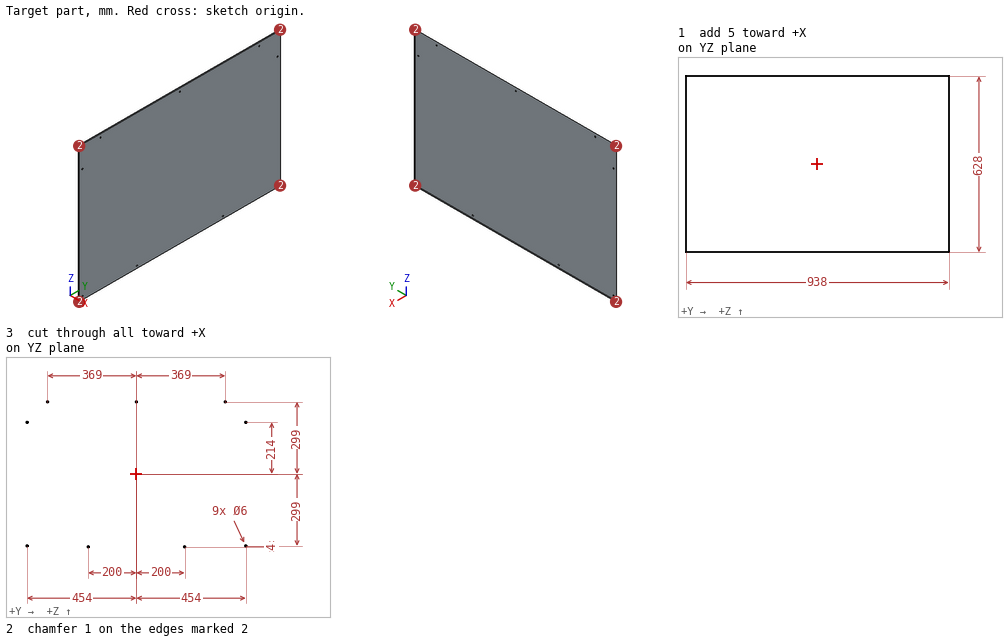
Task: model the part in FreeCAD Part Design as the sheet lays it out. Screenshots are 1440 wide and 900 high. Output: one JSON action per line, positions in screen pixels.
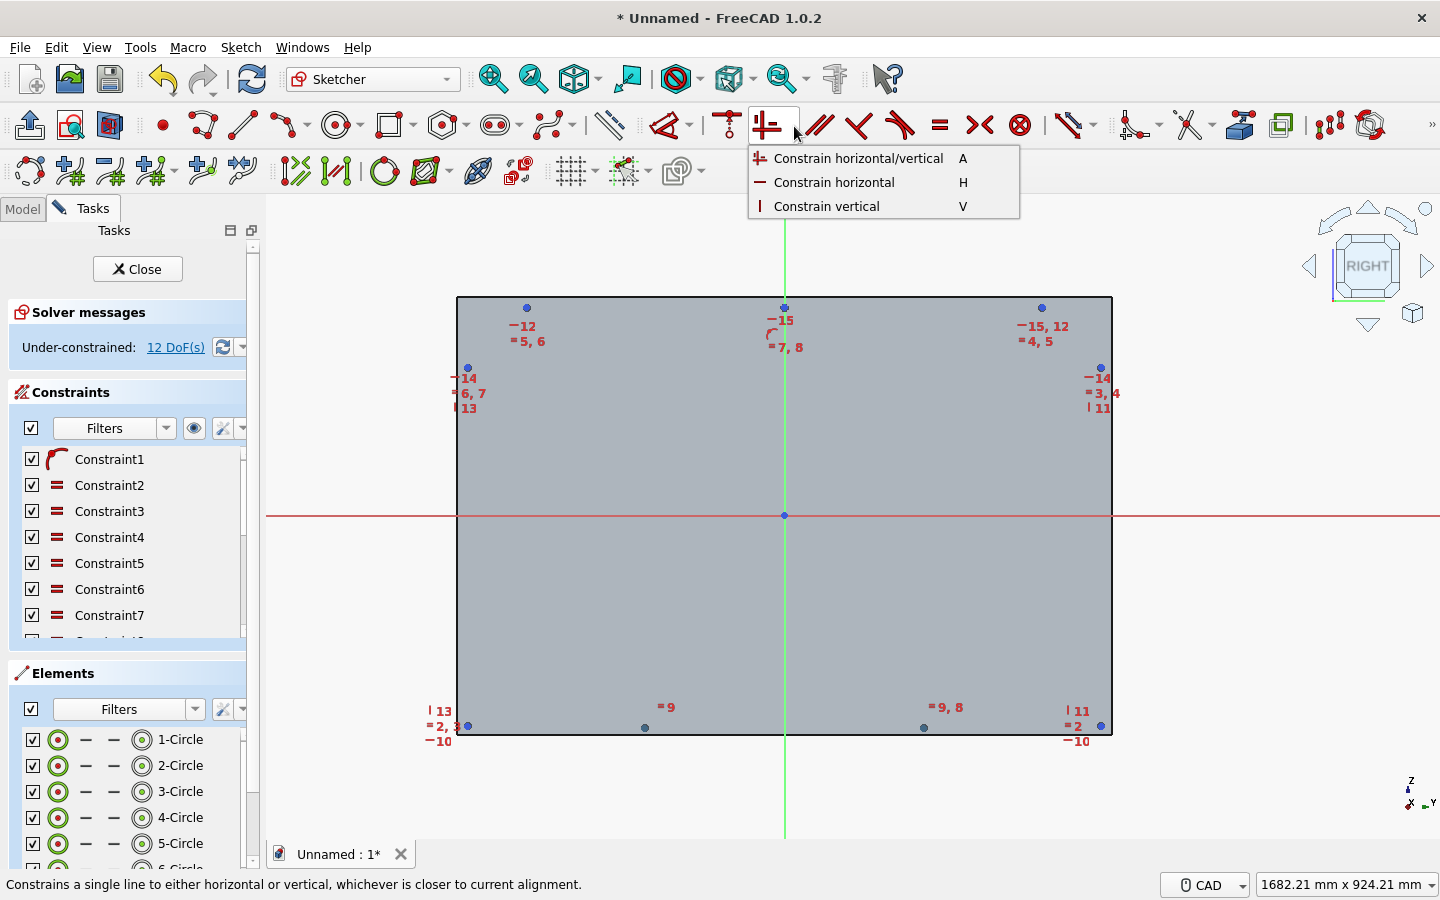
{"action": "left_click", "coordinate": [884, 182]}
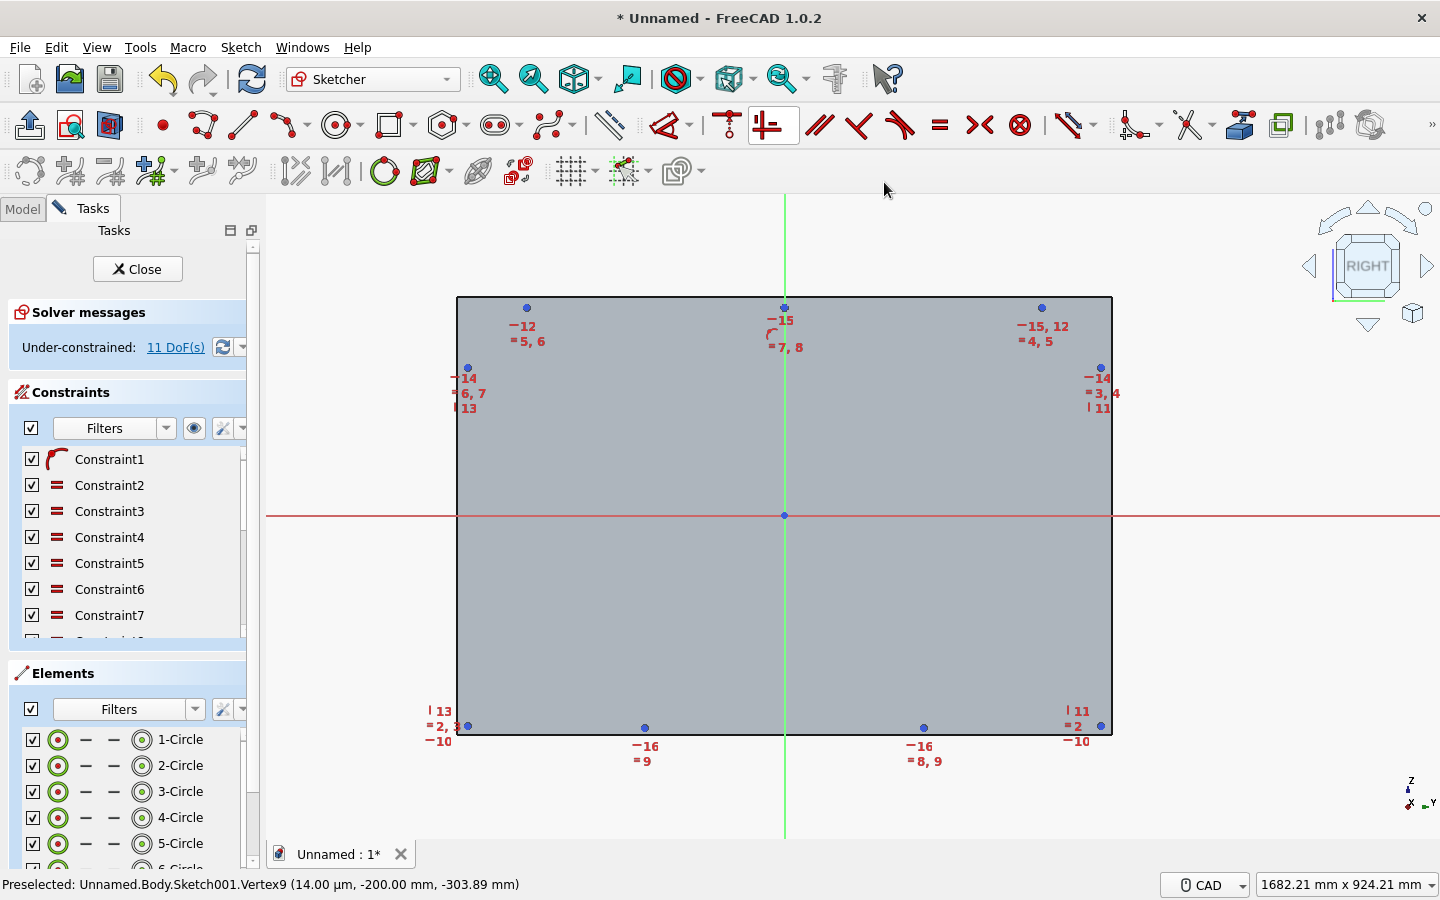
{"action": "left_click", "coordinate": [664, 126]}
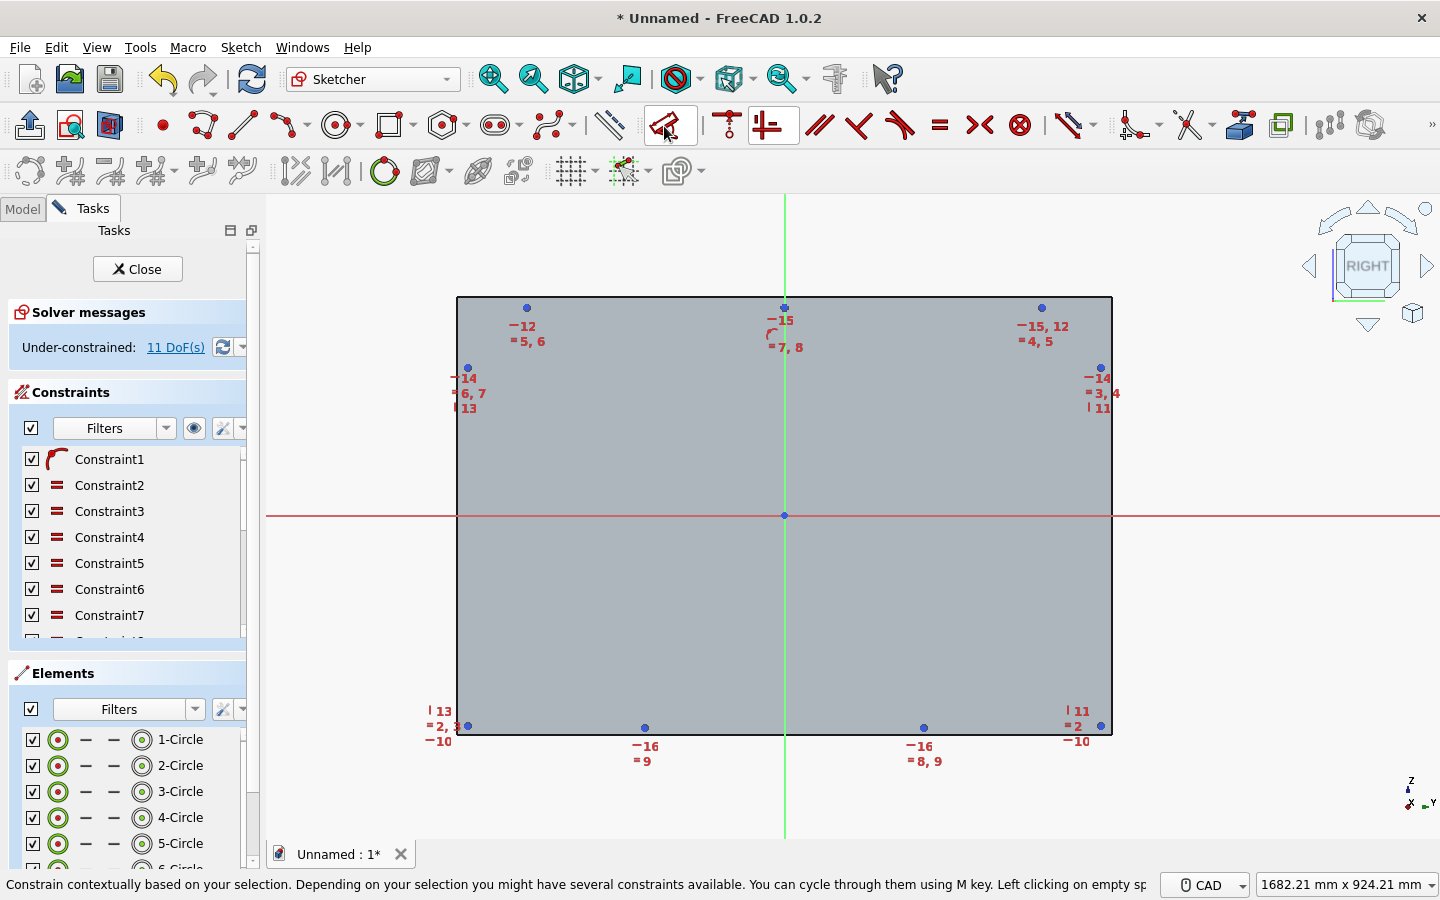
{"action": "scroll", "coordinate": [1101, 723], "scroll_direction": "up", "scroll_amount": 12}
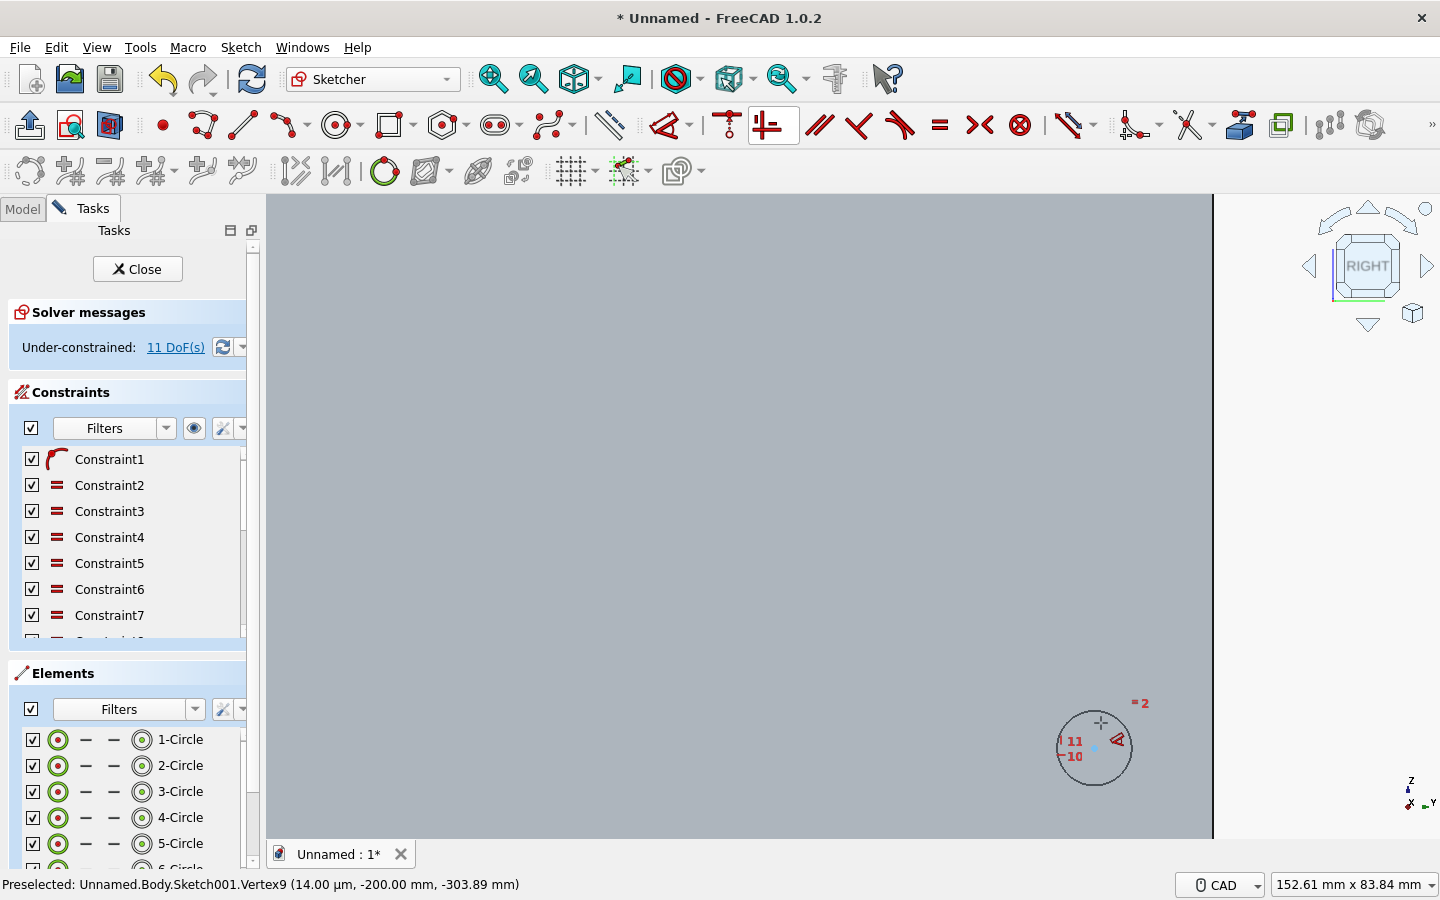
{"action": "left_click", "coordinate": [1095, 711]}
{"action": "left_click", "coordinate": [1095, 679]}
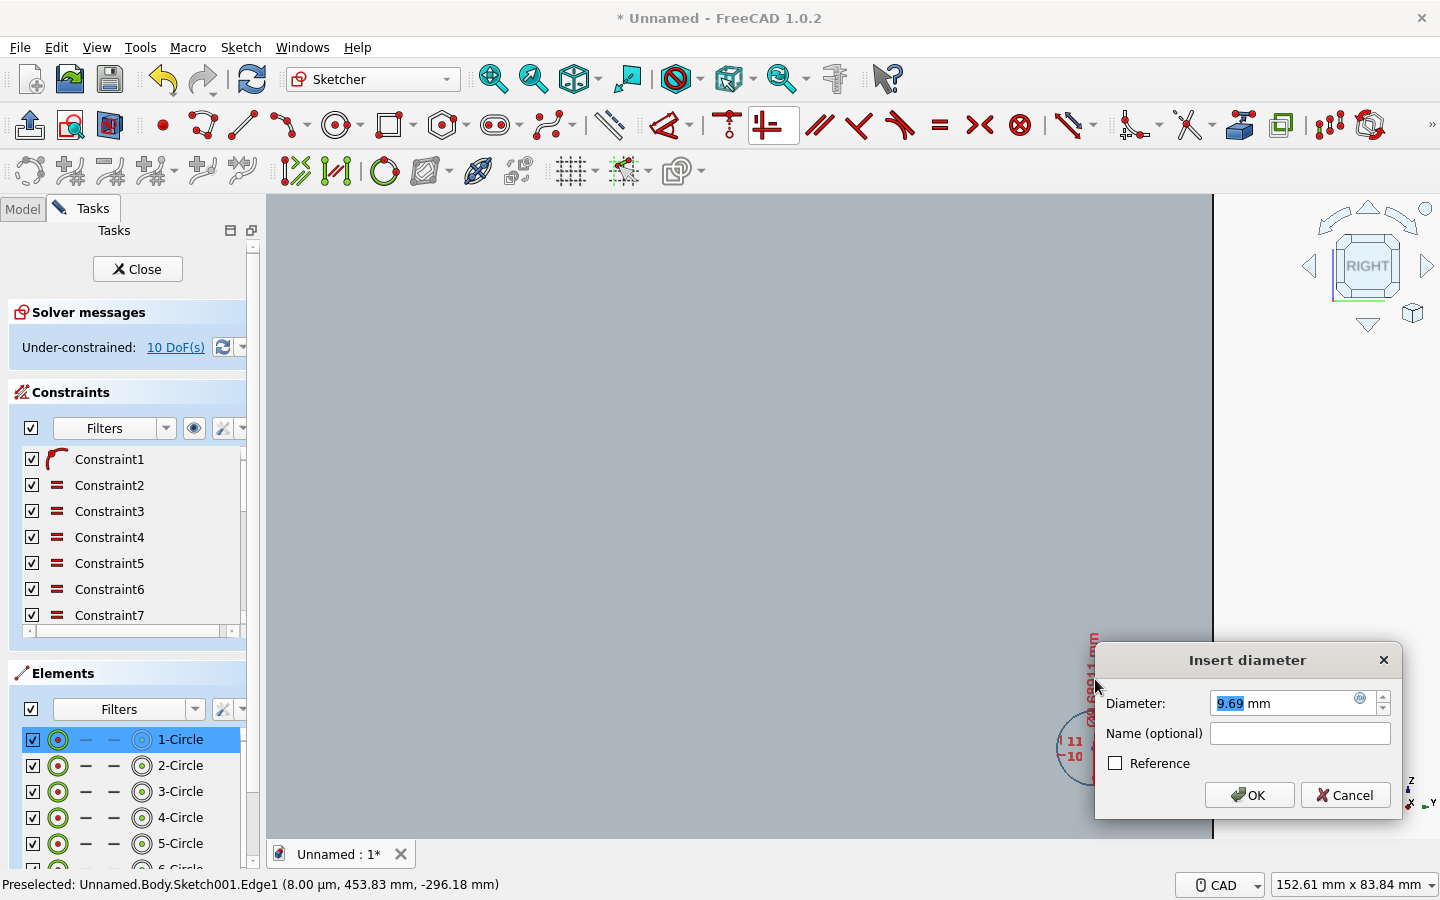
{"action": "type", "text": "6"}
{"action": "key", "text": "Return"}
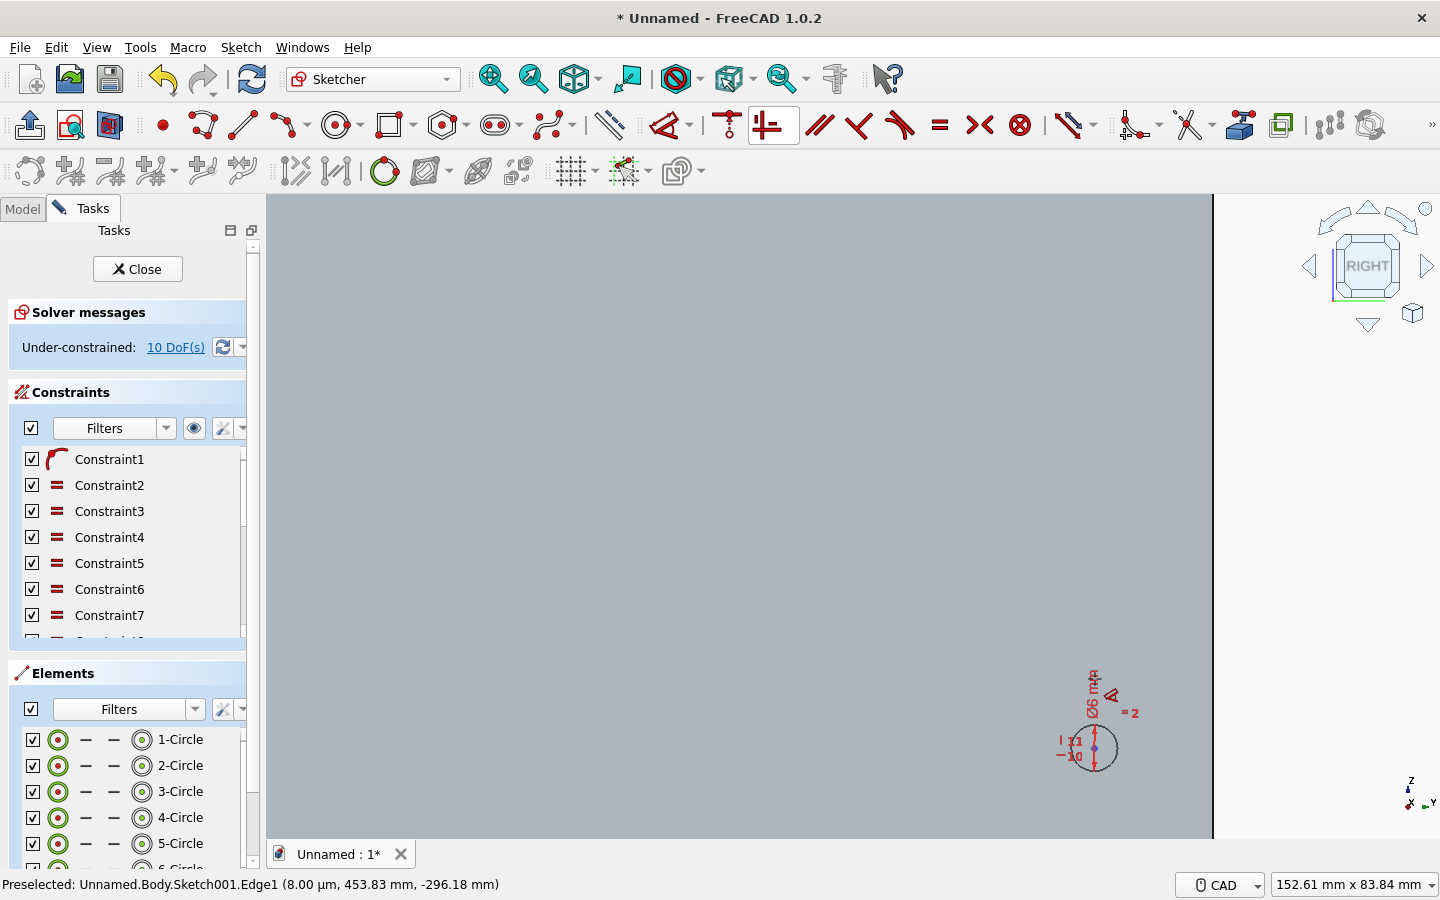
{"action": "scroll", "coordinate": [1094, 748], "scroll_direction": "up", "scroll_amount": 2}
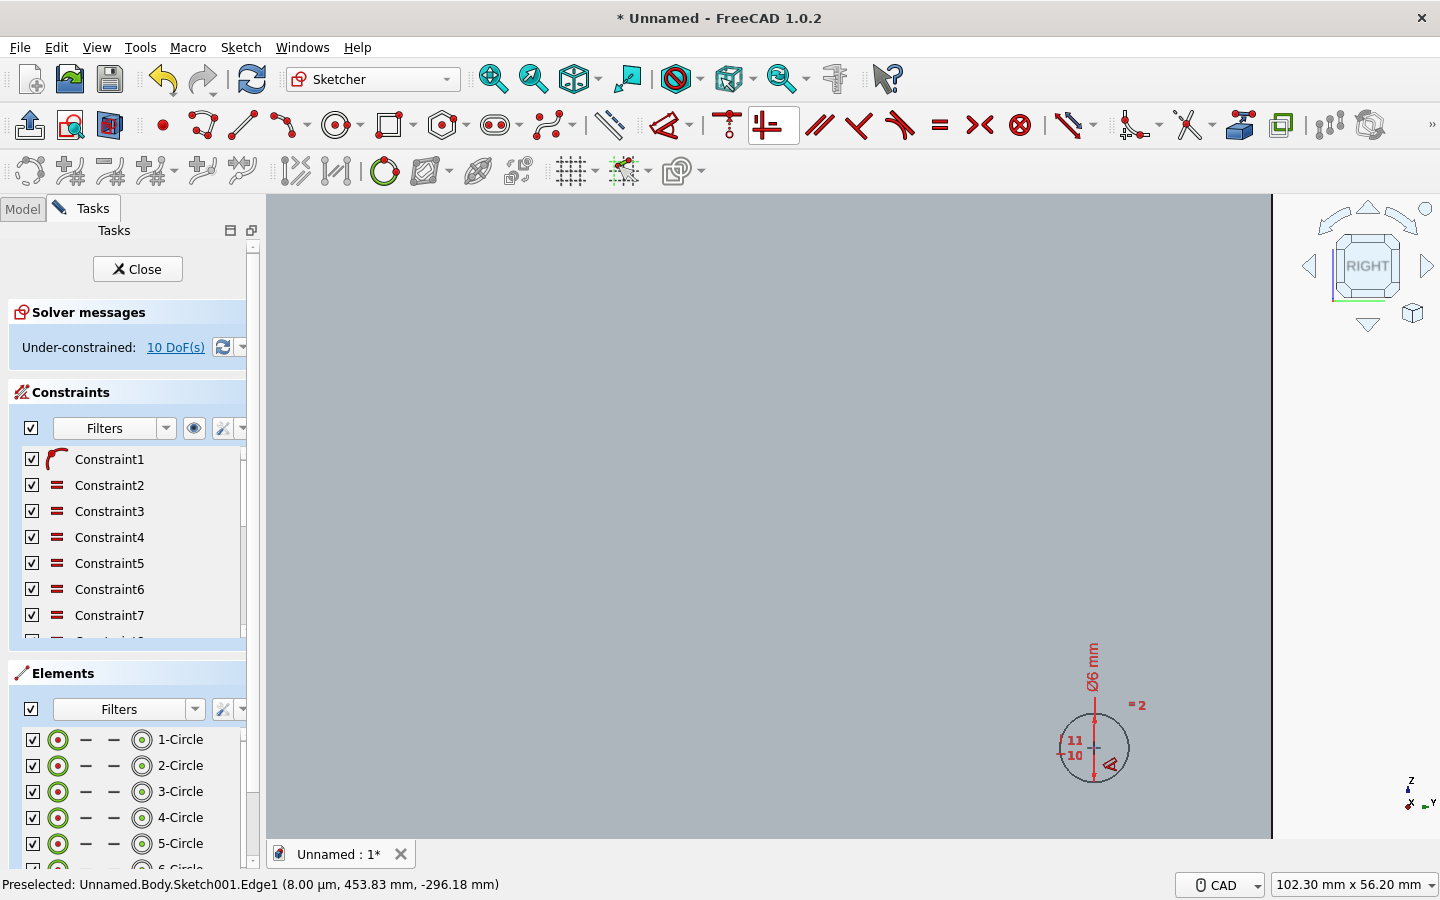
{"action": "left_click", "coordinate": [1094, 748]}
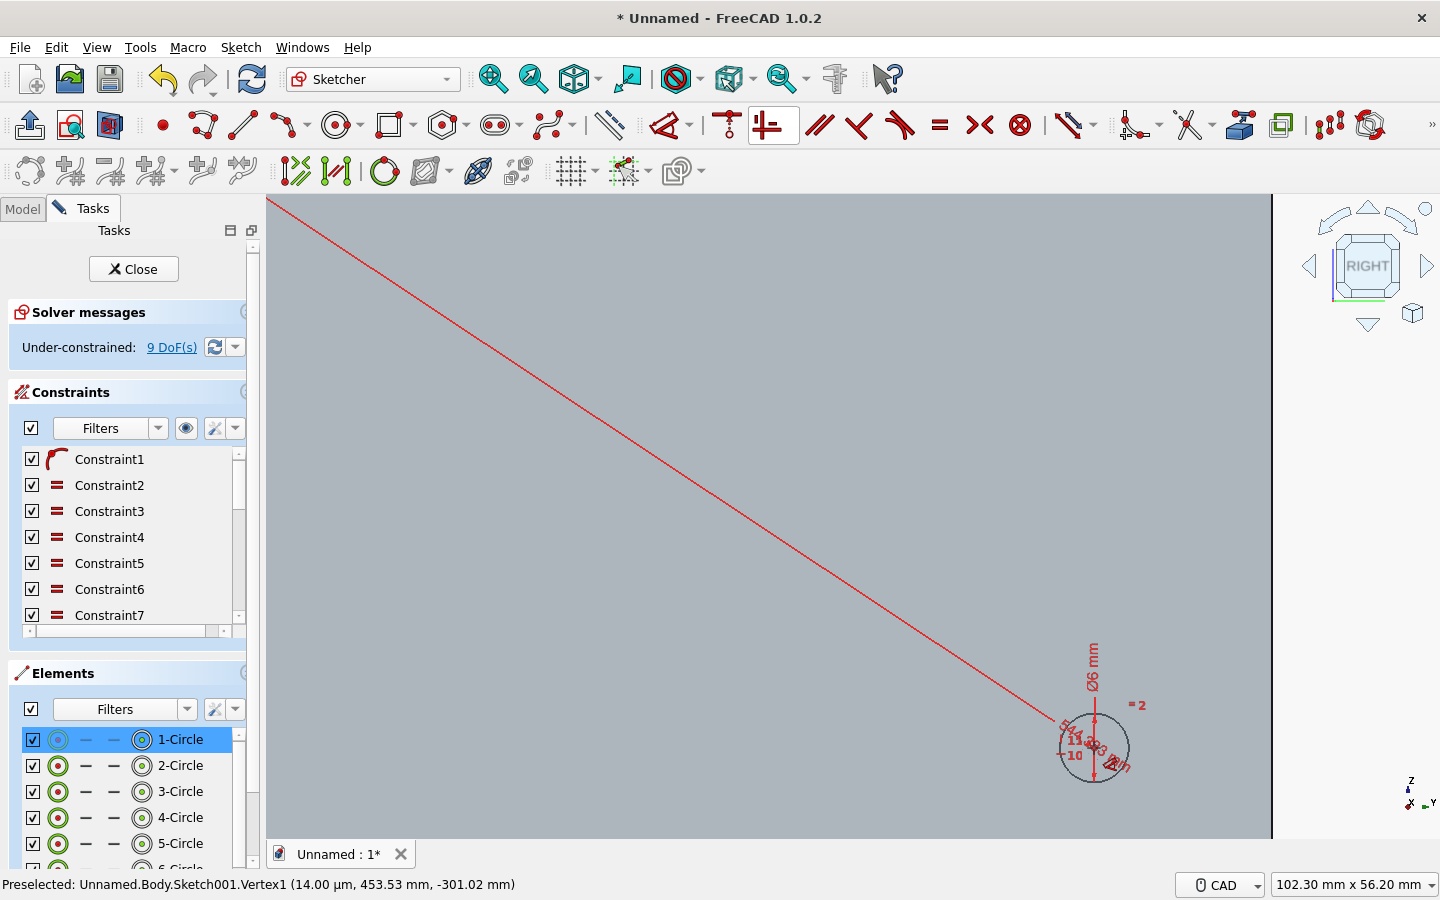
{"action": "scroll", "coordinate": [1101, 724], "scroll_direction": "down", "scroll_amount": 14}